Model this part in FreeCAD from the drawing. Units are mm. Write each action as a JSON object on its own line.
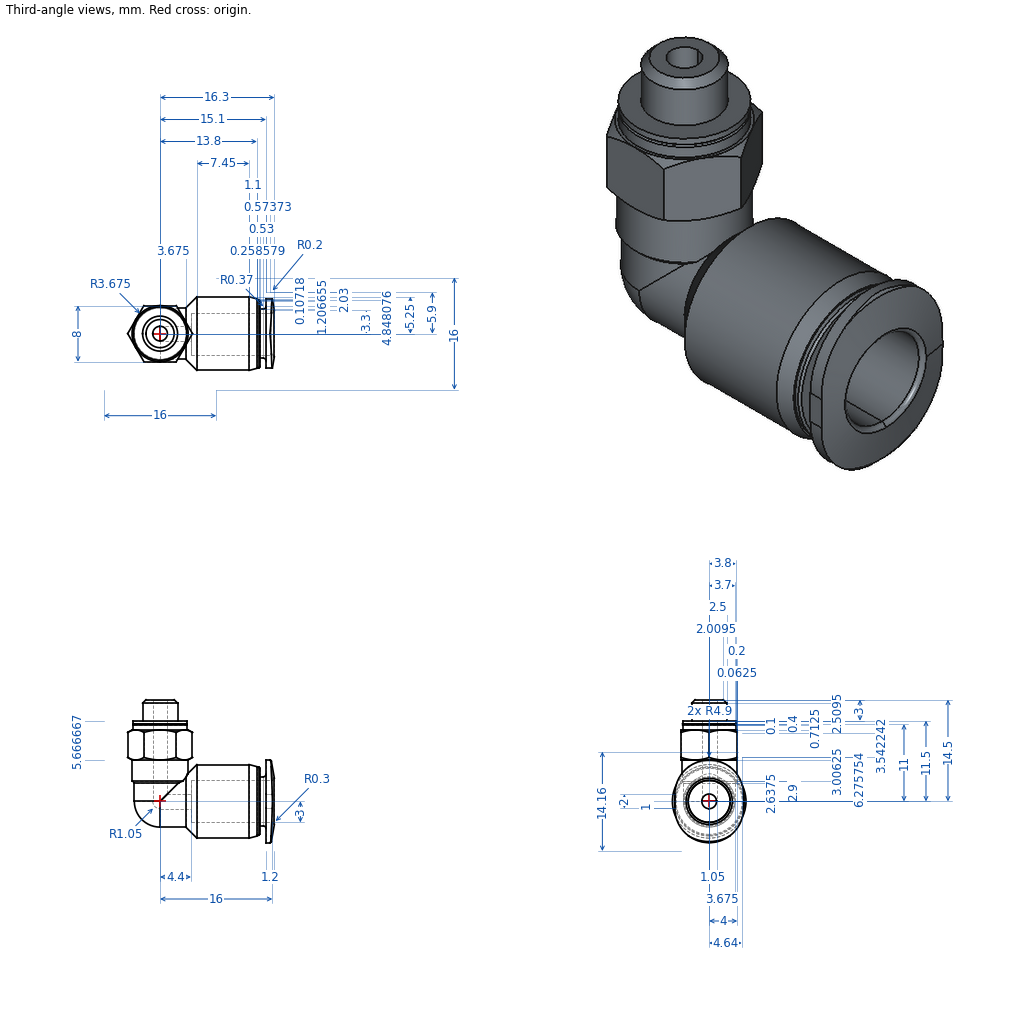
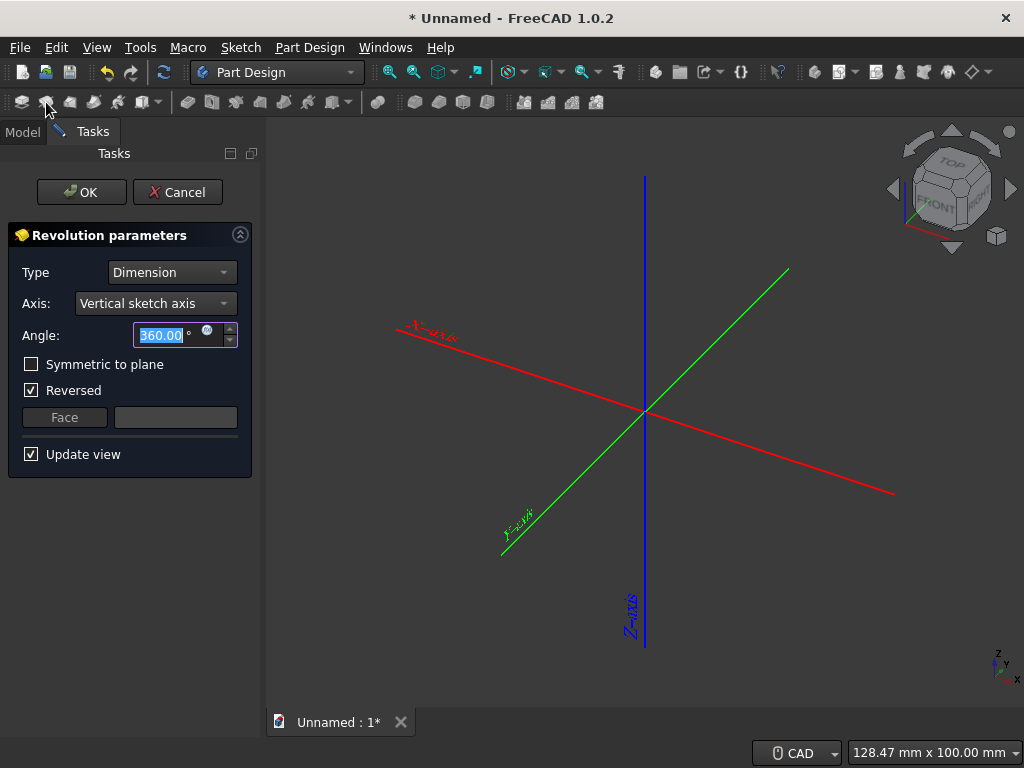
{"action": "left_click", "coordinate": [156, 304]}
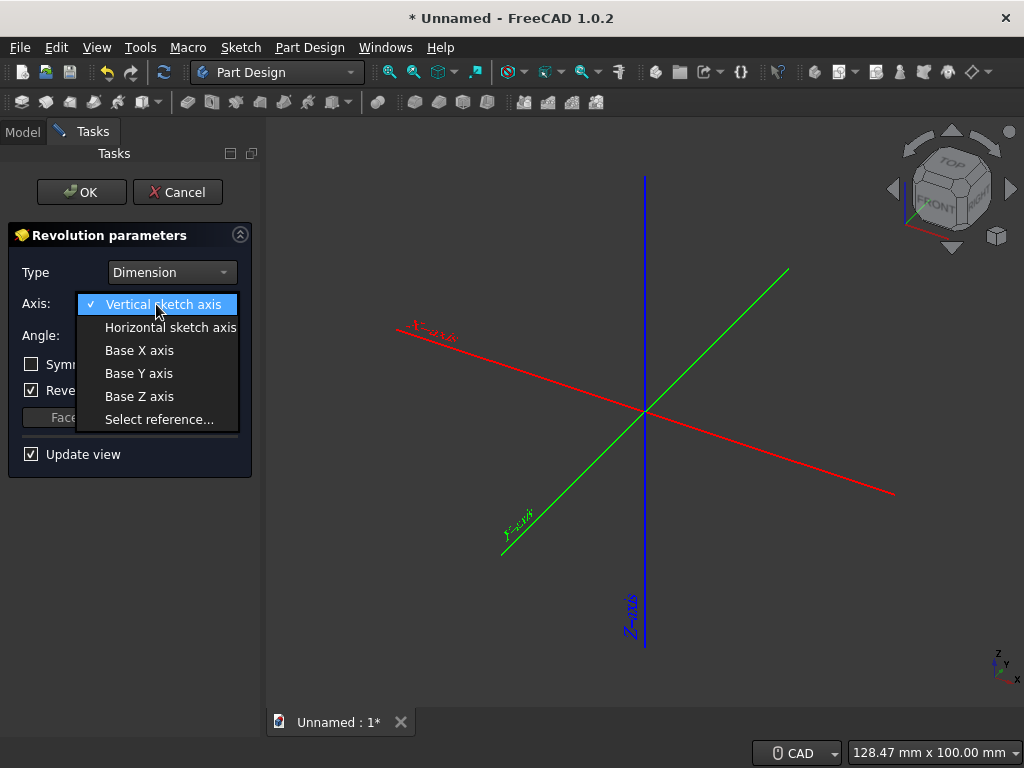
{"action": "left_click", "coordinate": [156, 328]}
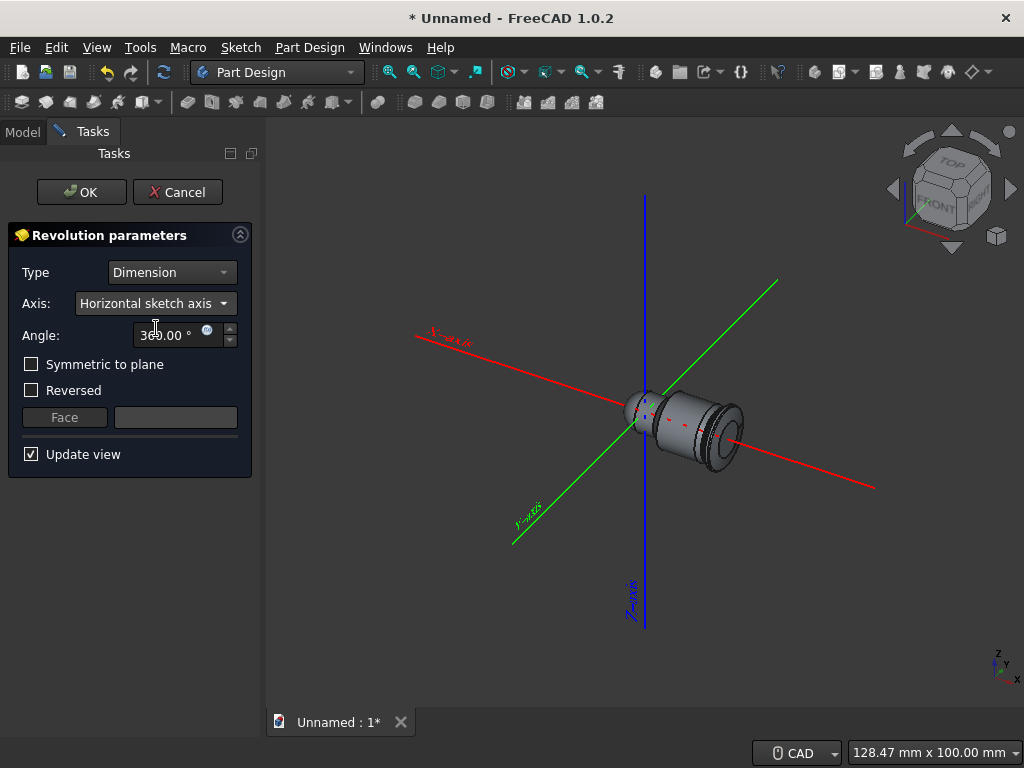
{"action": "left_click", "coordinate": [82, 192]}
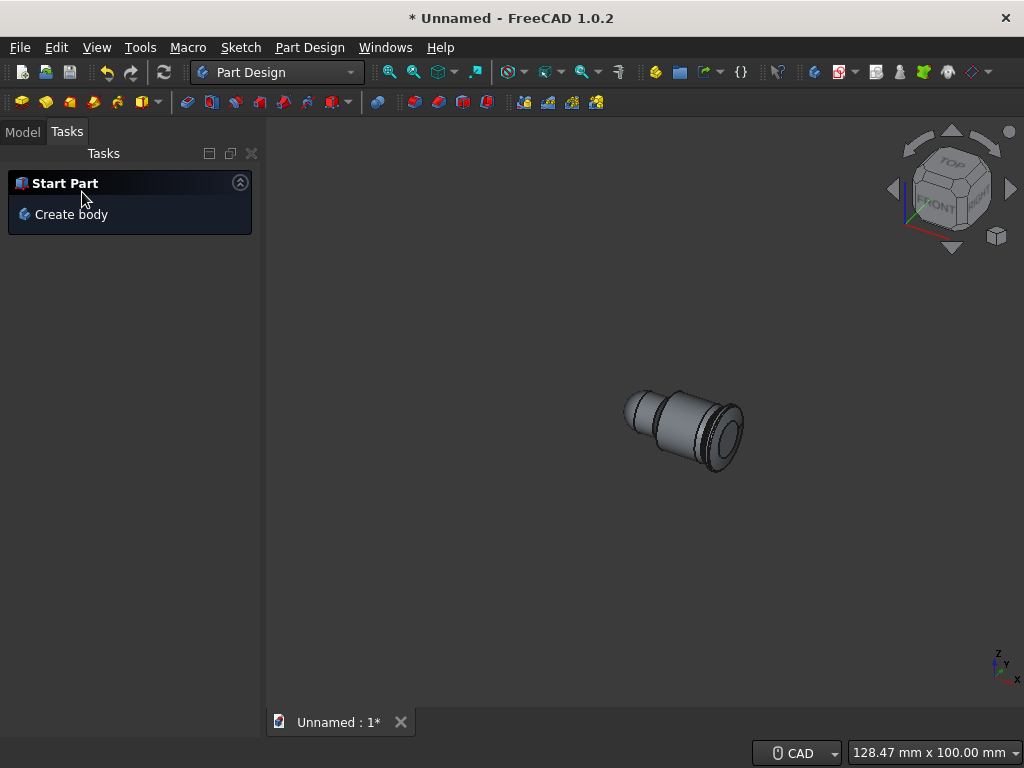
{"action": "left_click", "coordinate": [390, 72]}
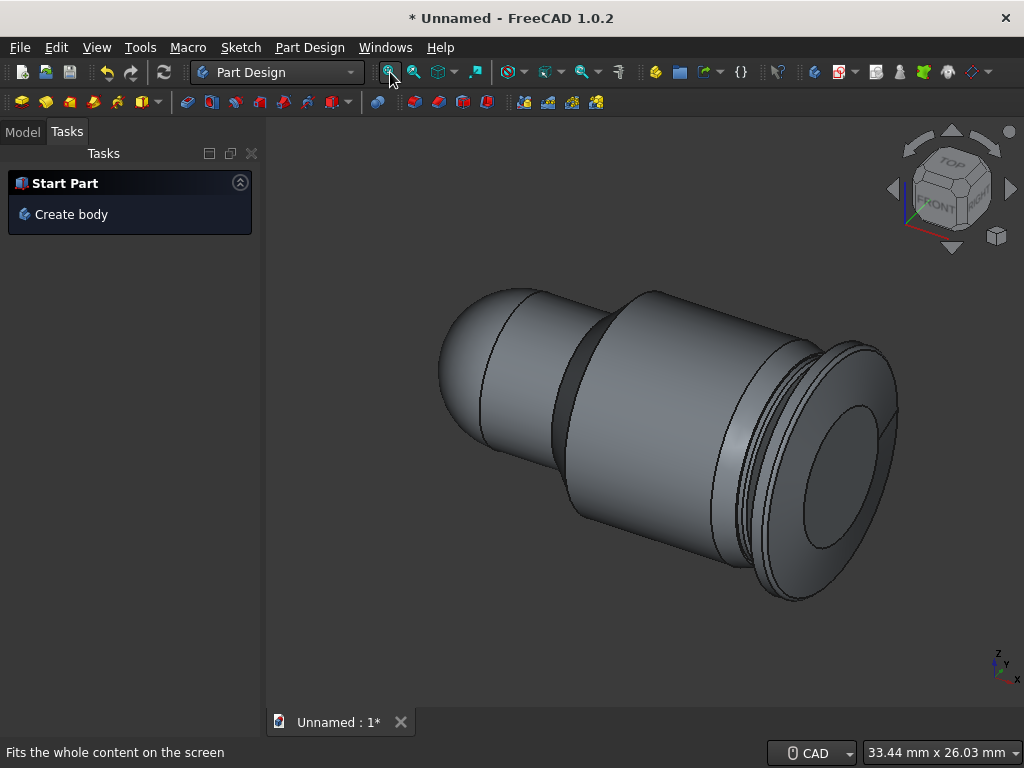
{"action": "left_click", "coordinate": [840, 72]}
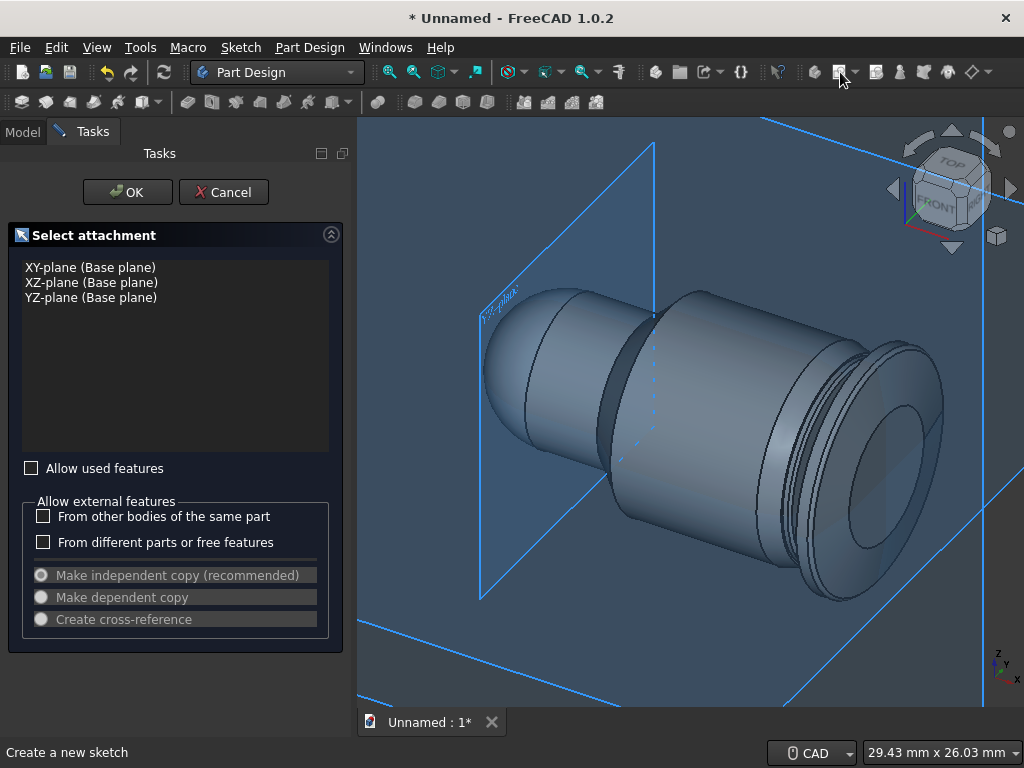
{"action": "left_click", "coordinate": [82, 298]}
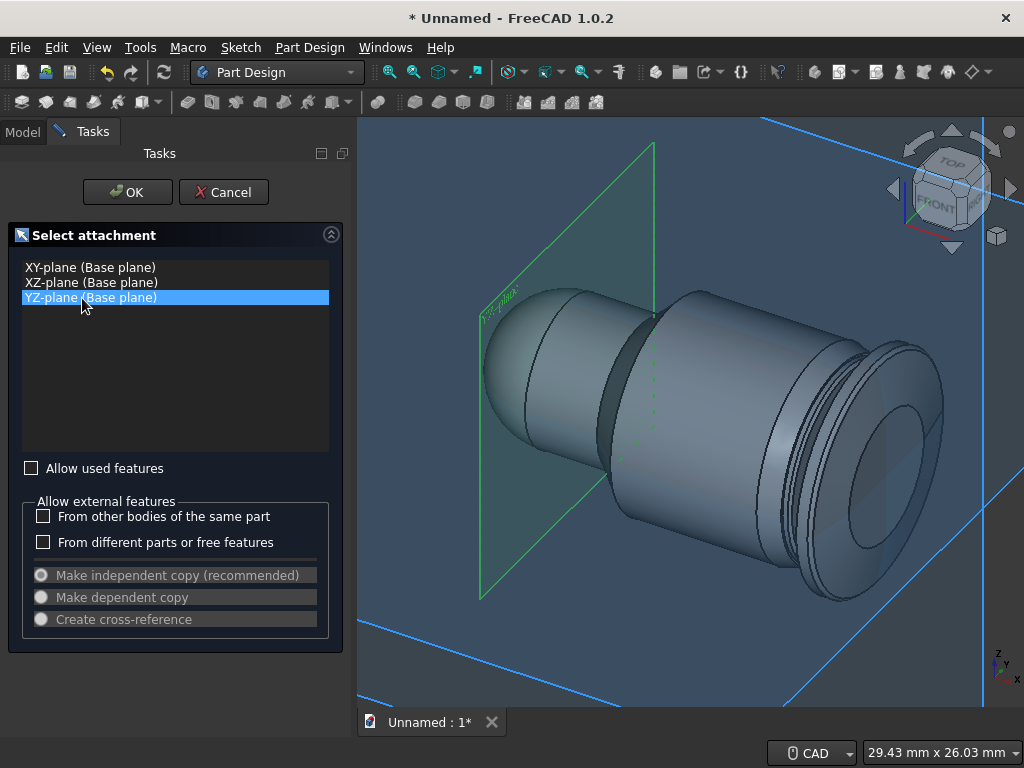
{"action": "left_click", "coordinate": [128, 192]}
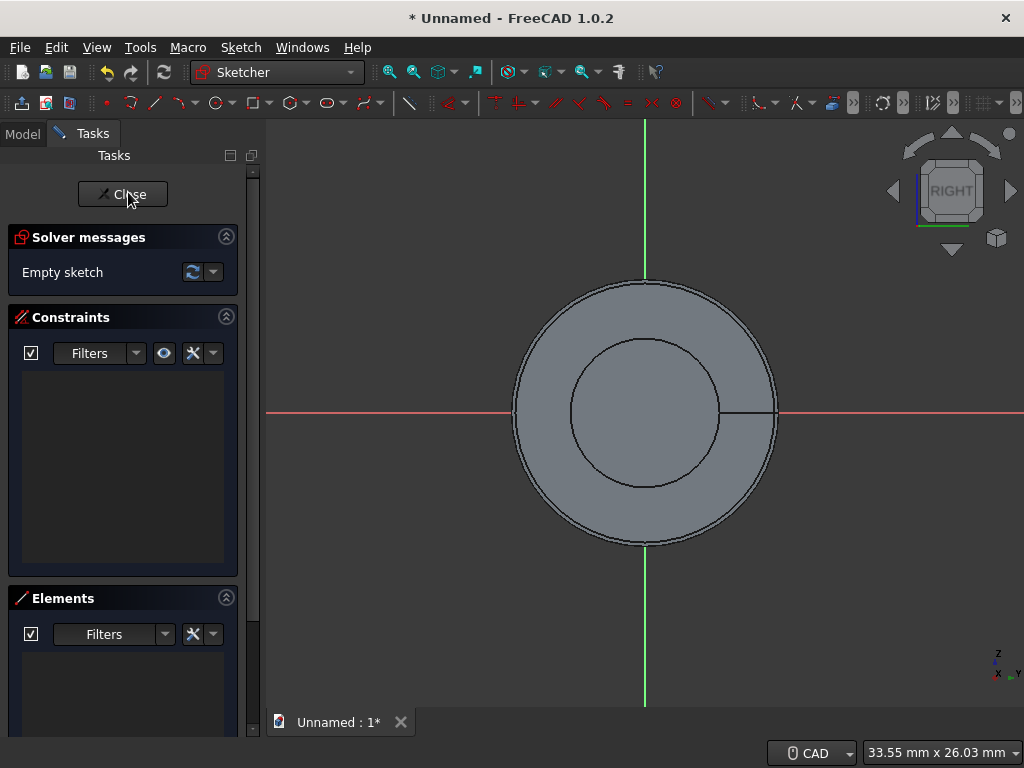
{"action": "left_click", "coordinate": [70, 104]}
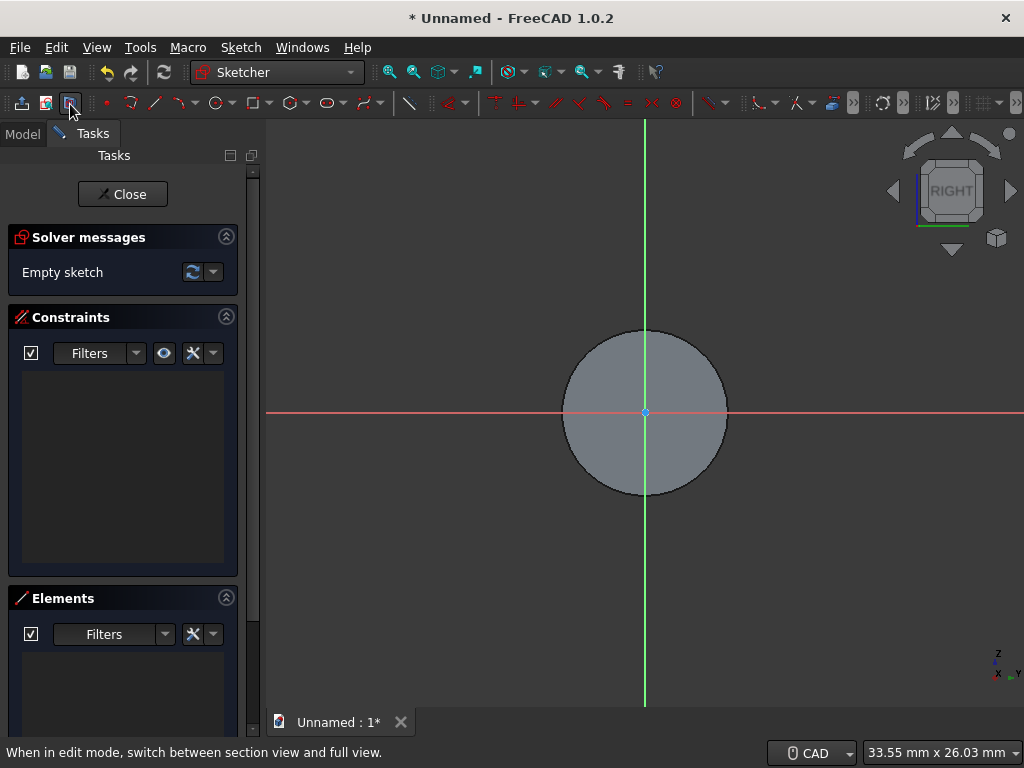
{"action": "scroll", "coordinate": [294, 679], "scroll_direction": "down", "scroll_amount": 1}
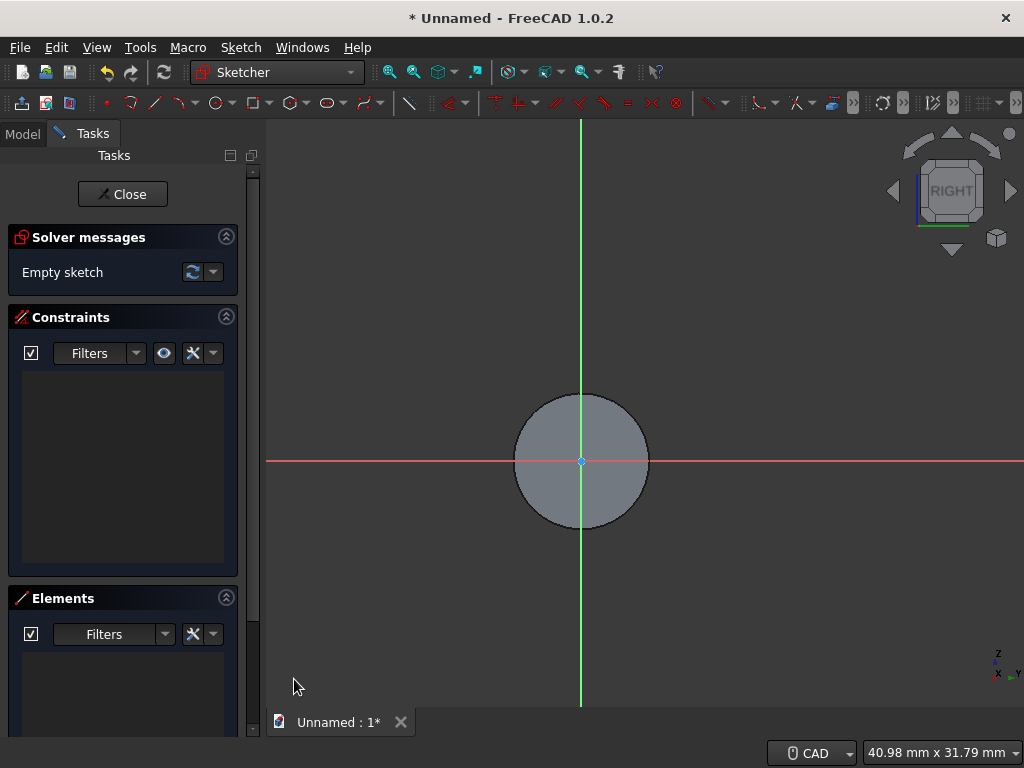
{"action": "scroll", "coordinate": [682, 285], "scroll_direction": "up", "scroll_amount": 3}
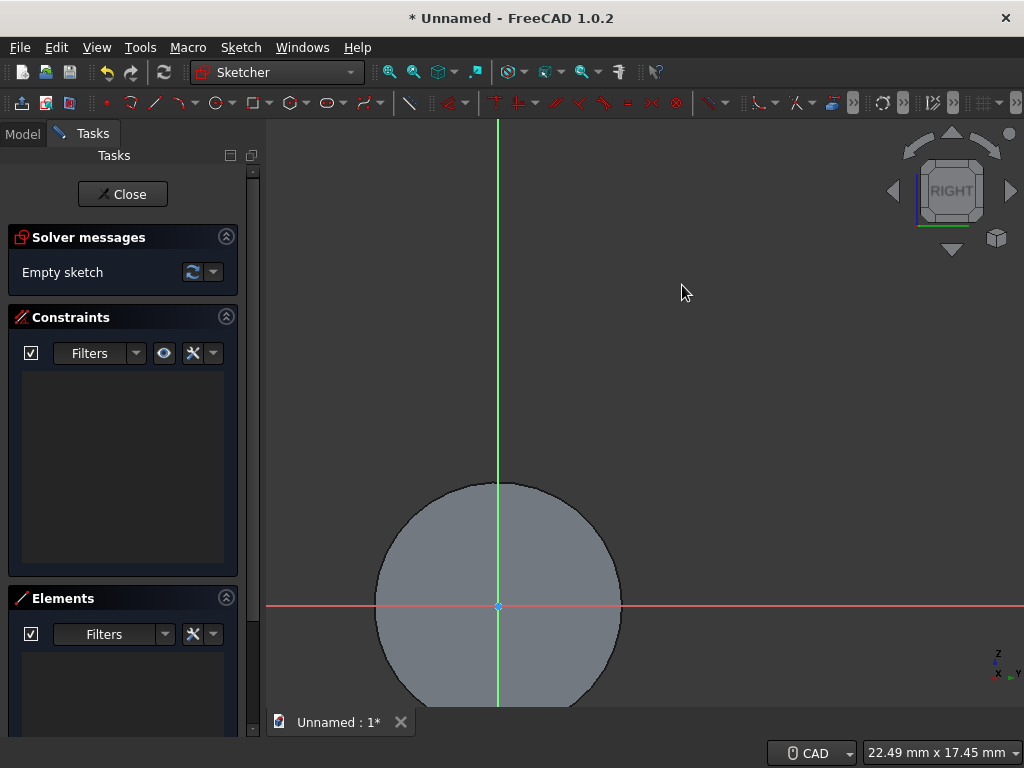
{"action": "left_click", "coordinate": [132, 104]}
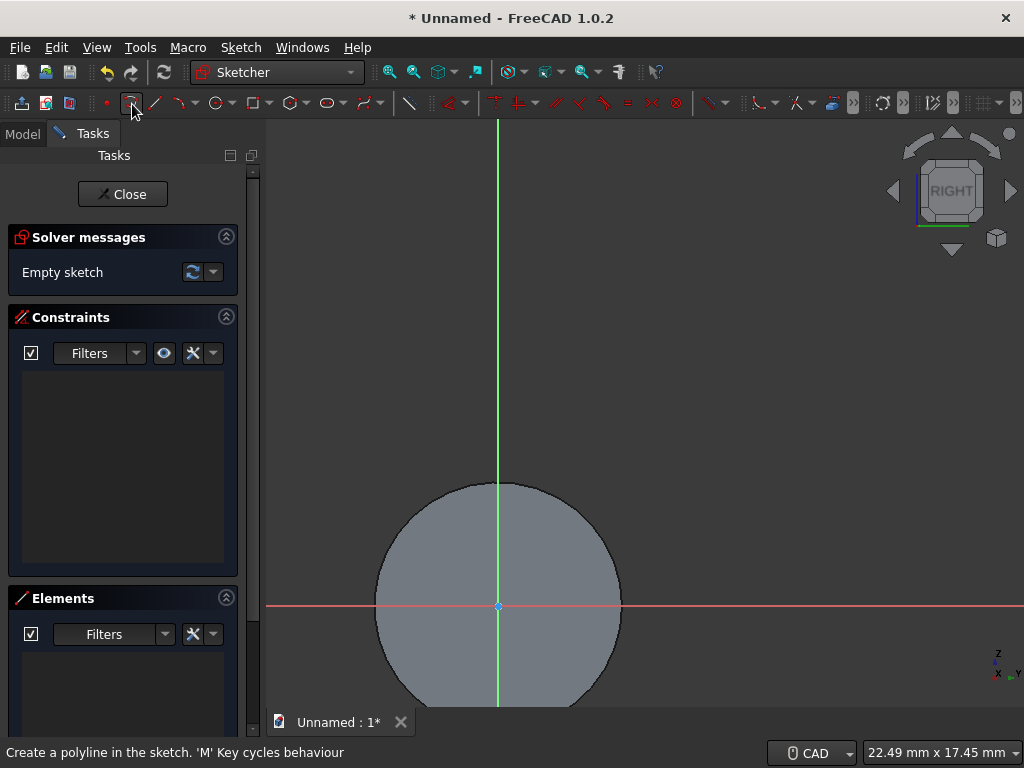
{"action": "left_click", "coordinate": [498, 606]}
{"action": "left_click", "coordinate": [622, 597]}
{"action": "left_click", "coordinate": [622, 517]}